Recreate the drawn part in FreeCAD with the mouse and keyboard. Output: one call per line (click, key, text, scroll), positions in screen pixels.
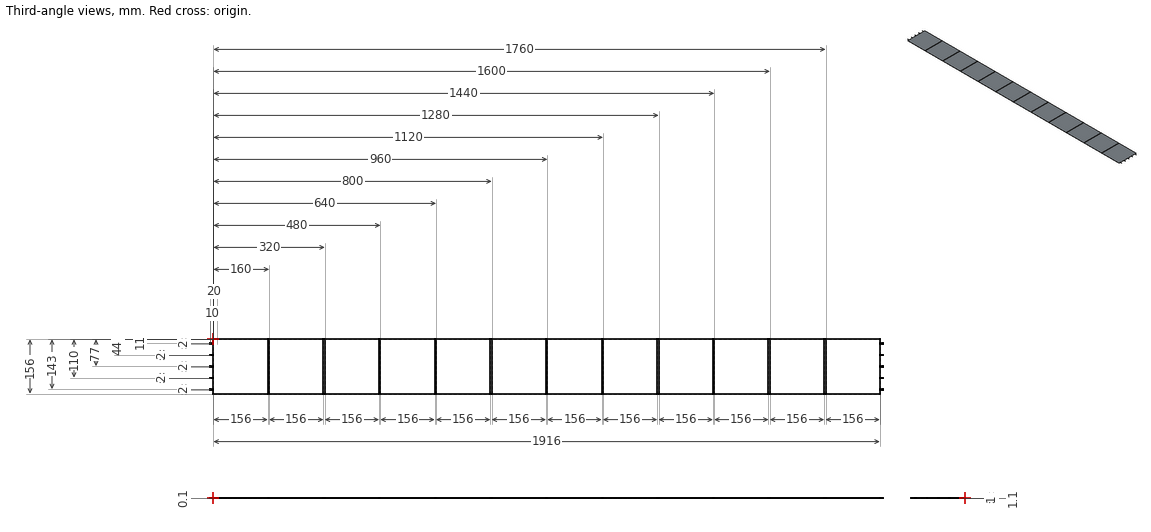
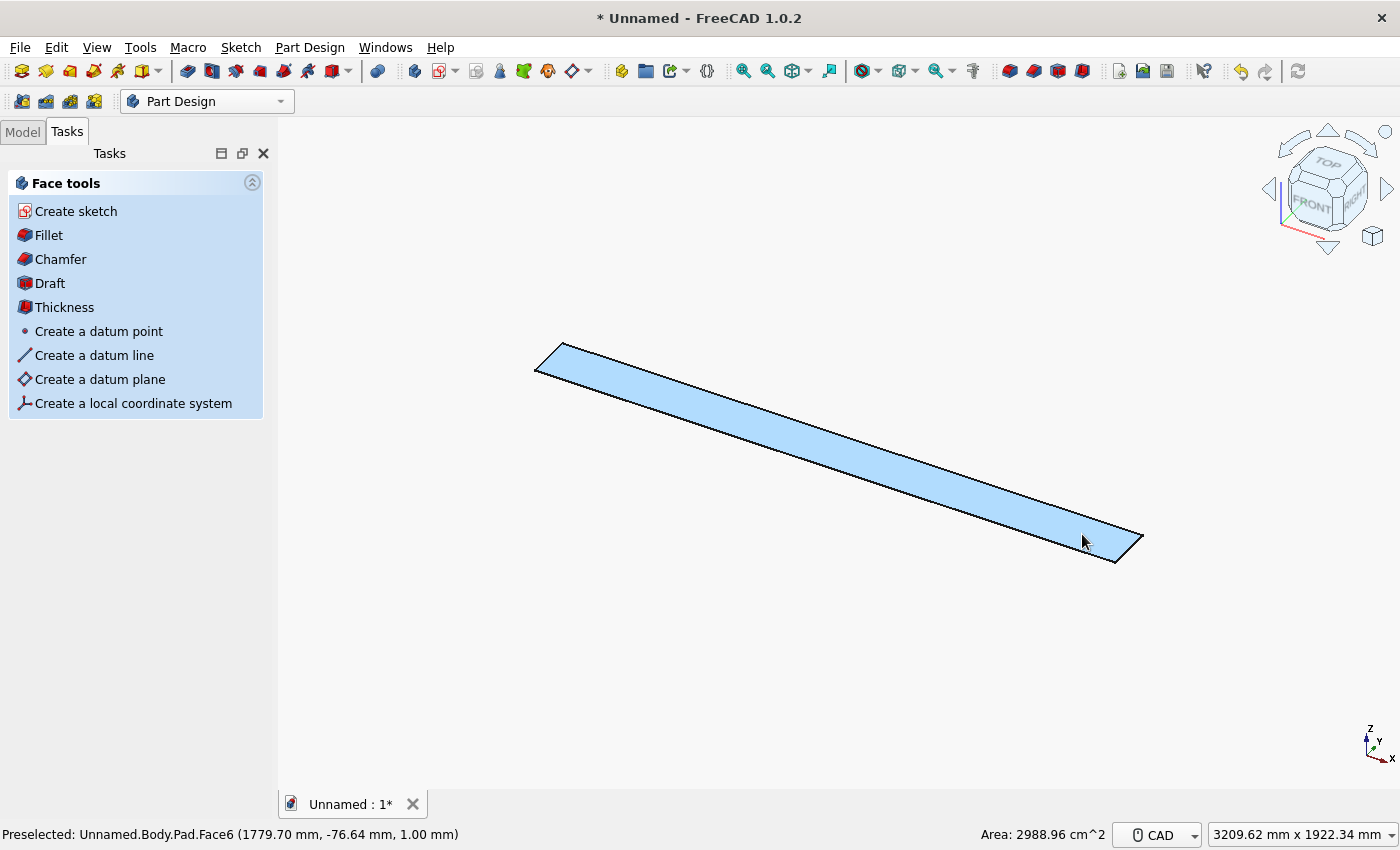
click(440, 72)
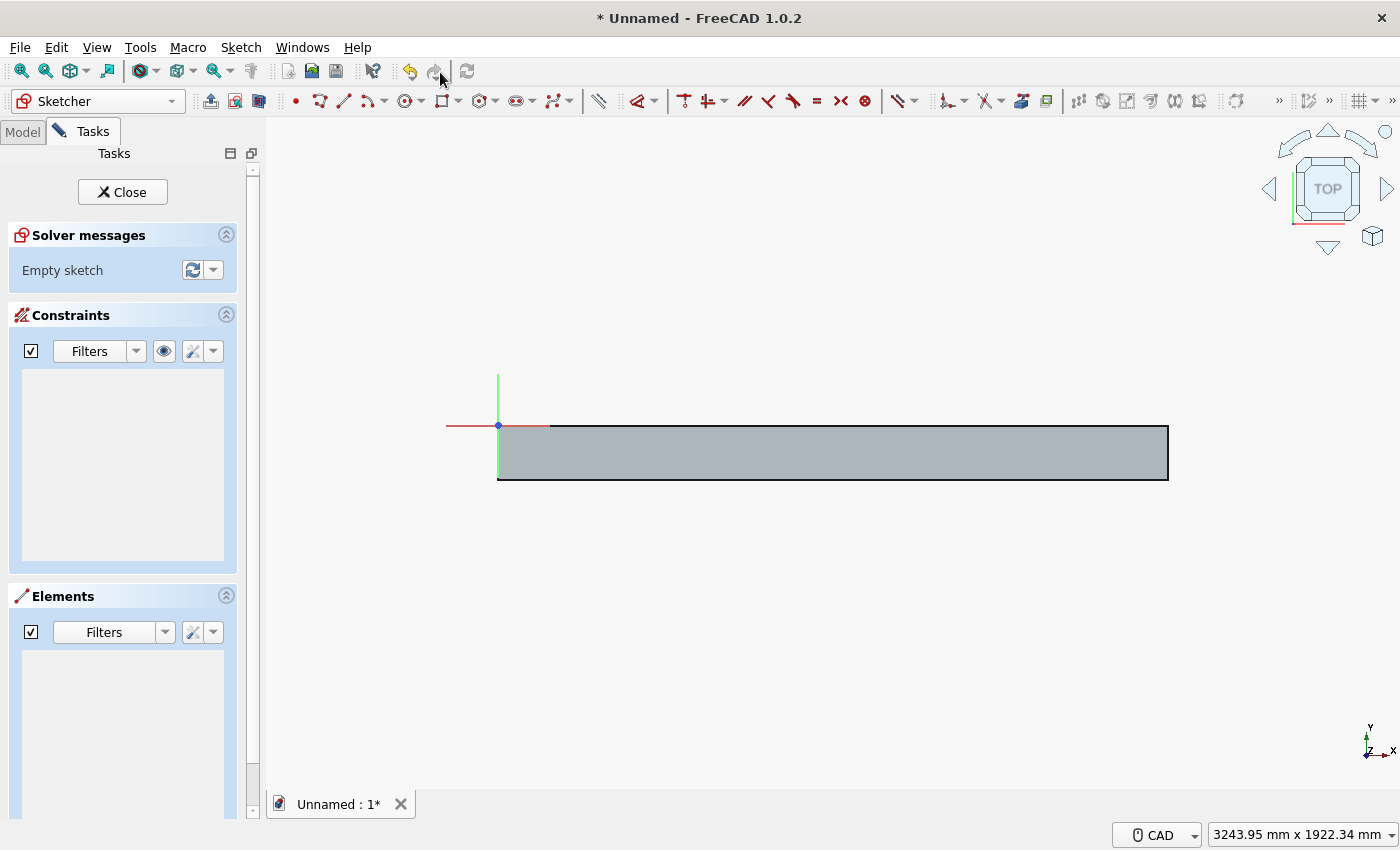
key(g)
key(r)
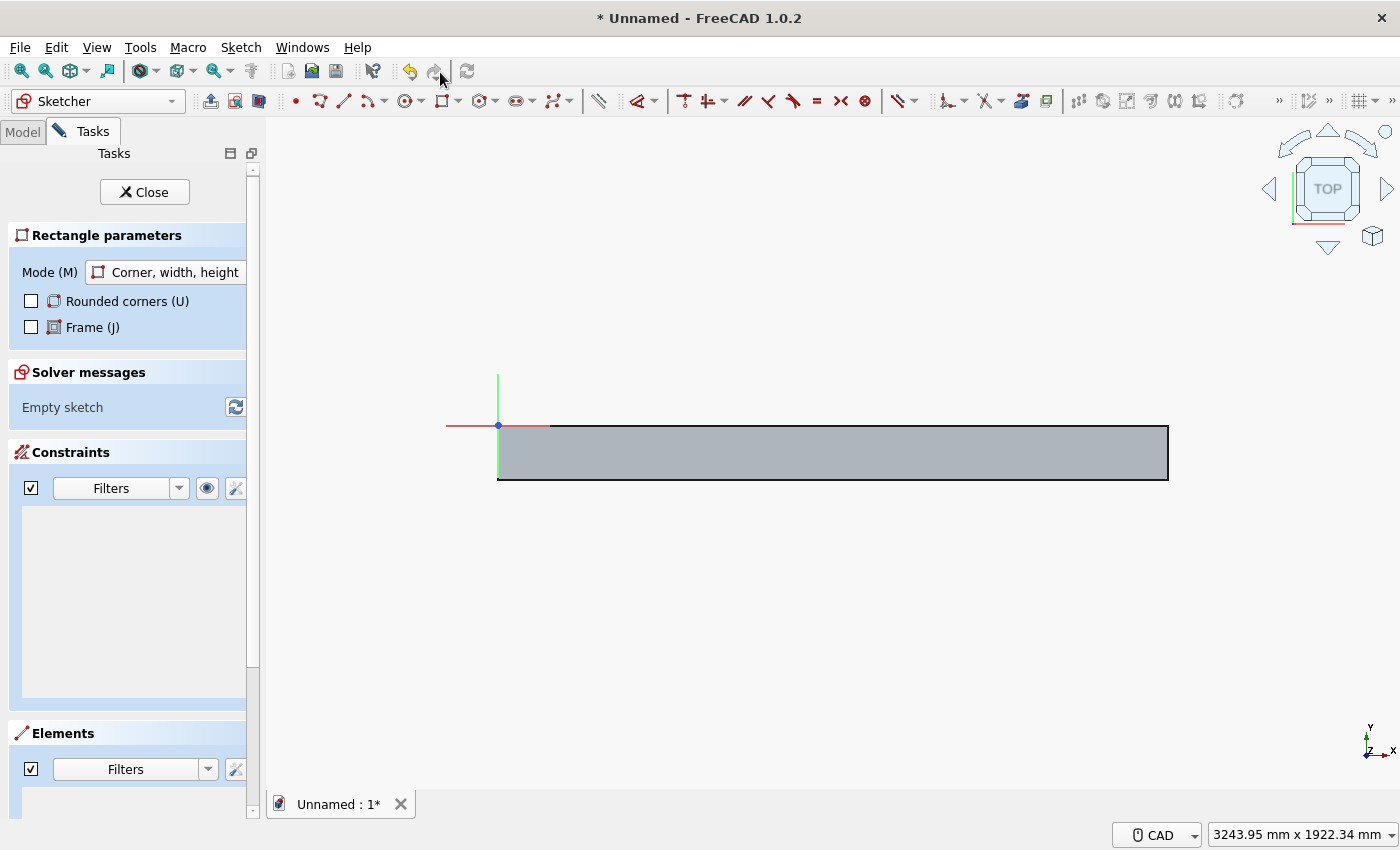
click(498, 426)
click(553, 480)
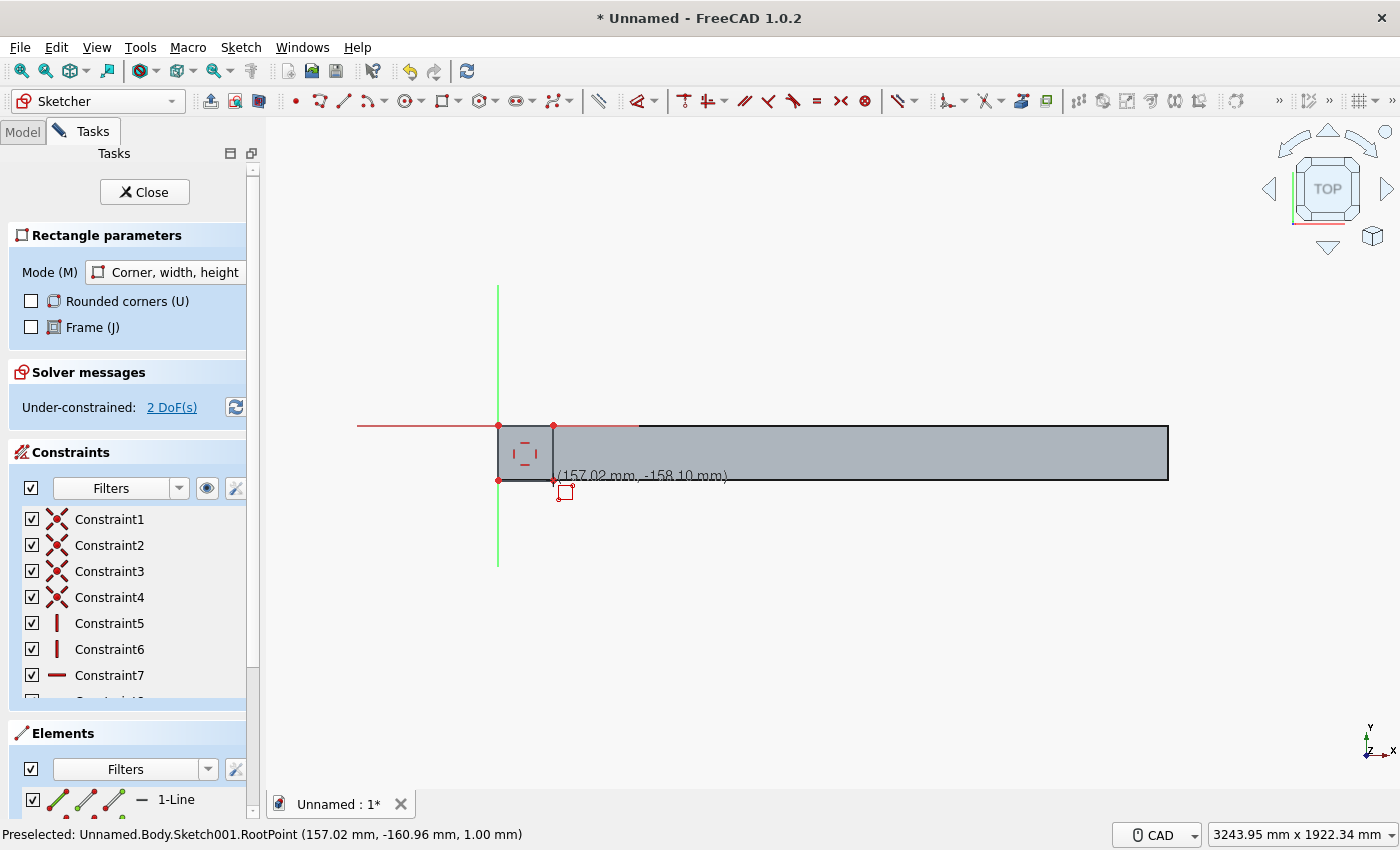
scroll(554, 426, up, 13)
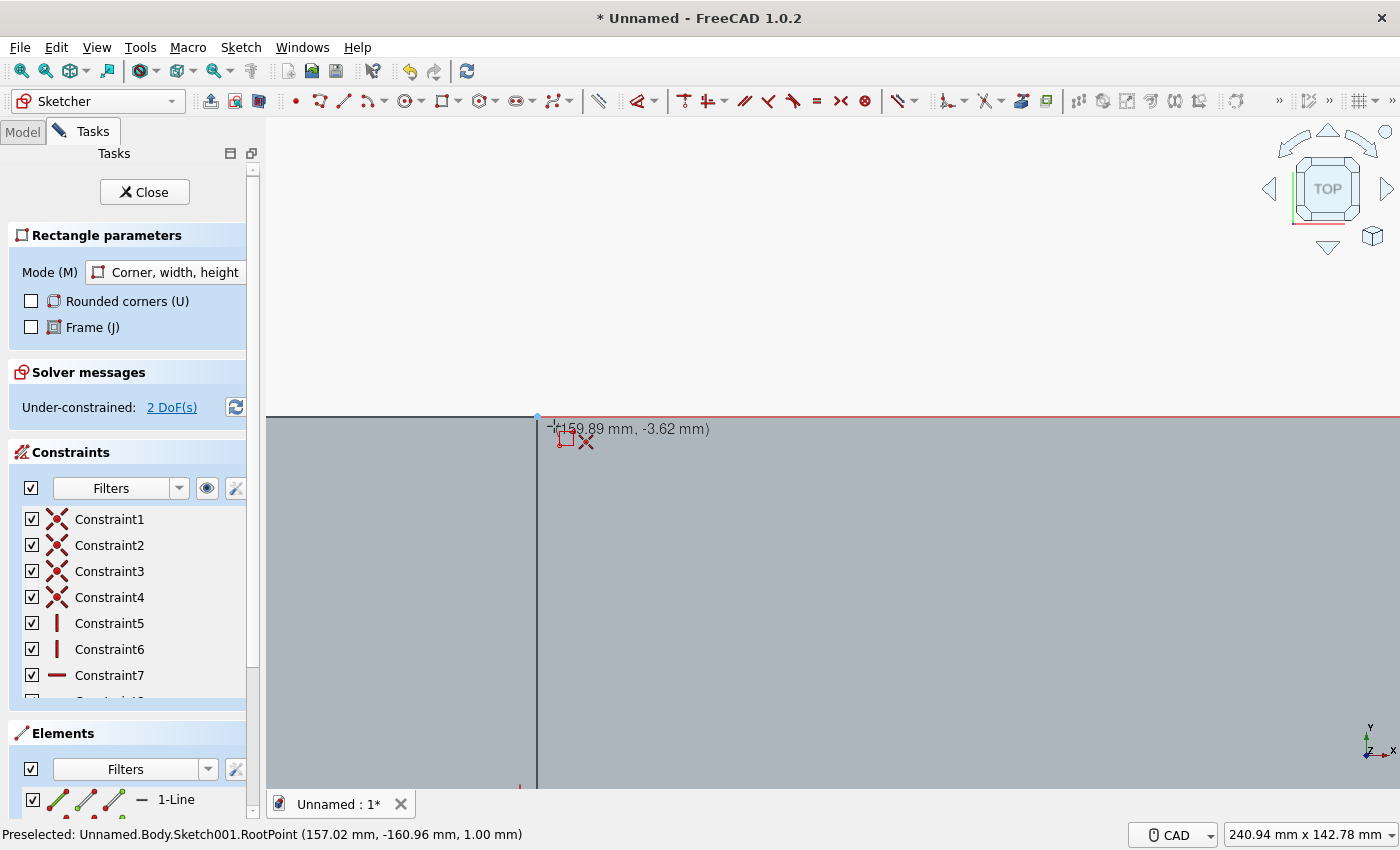
click(551, 417)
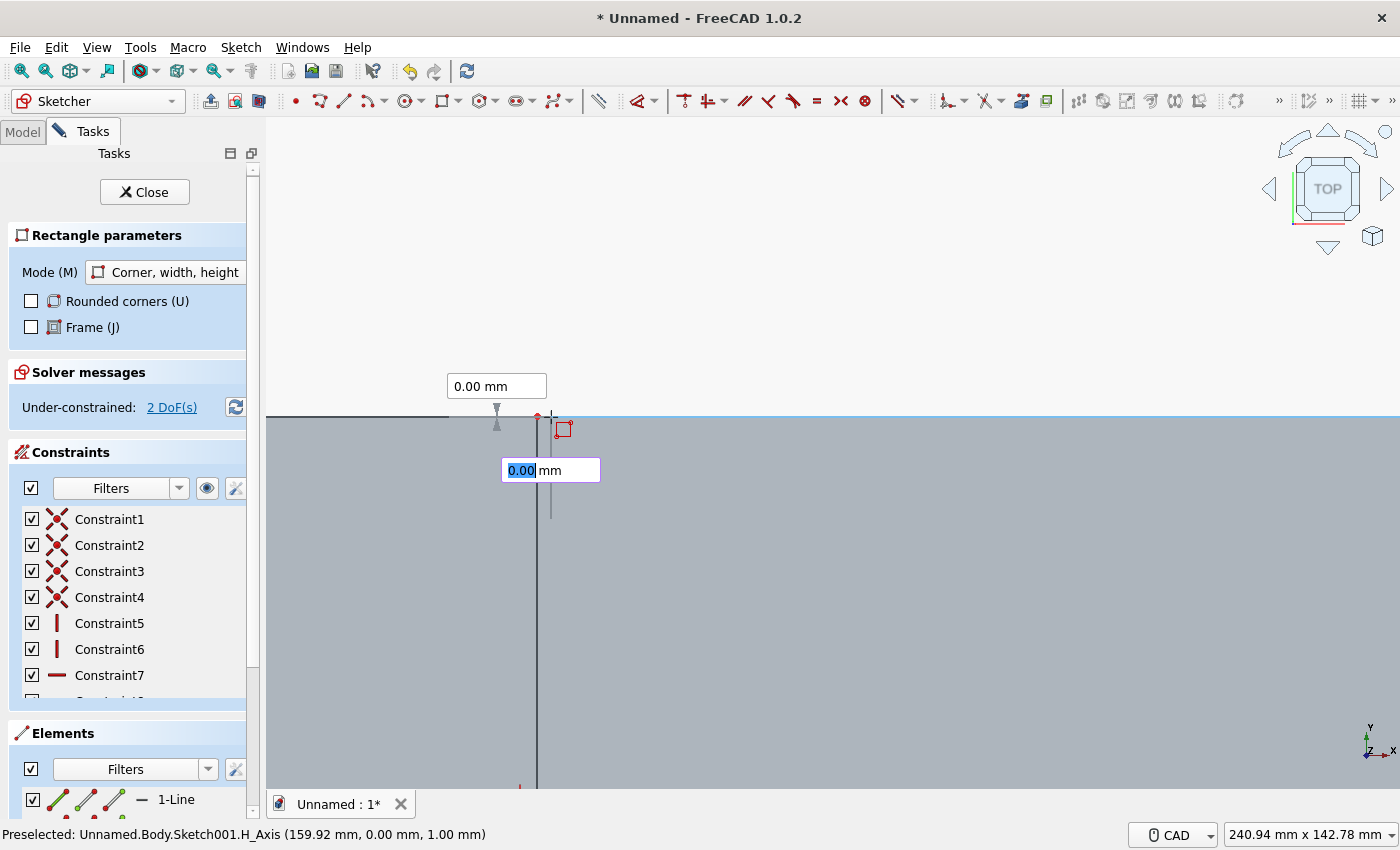
scroll(480, 426, down, 13)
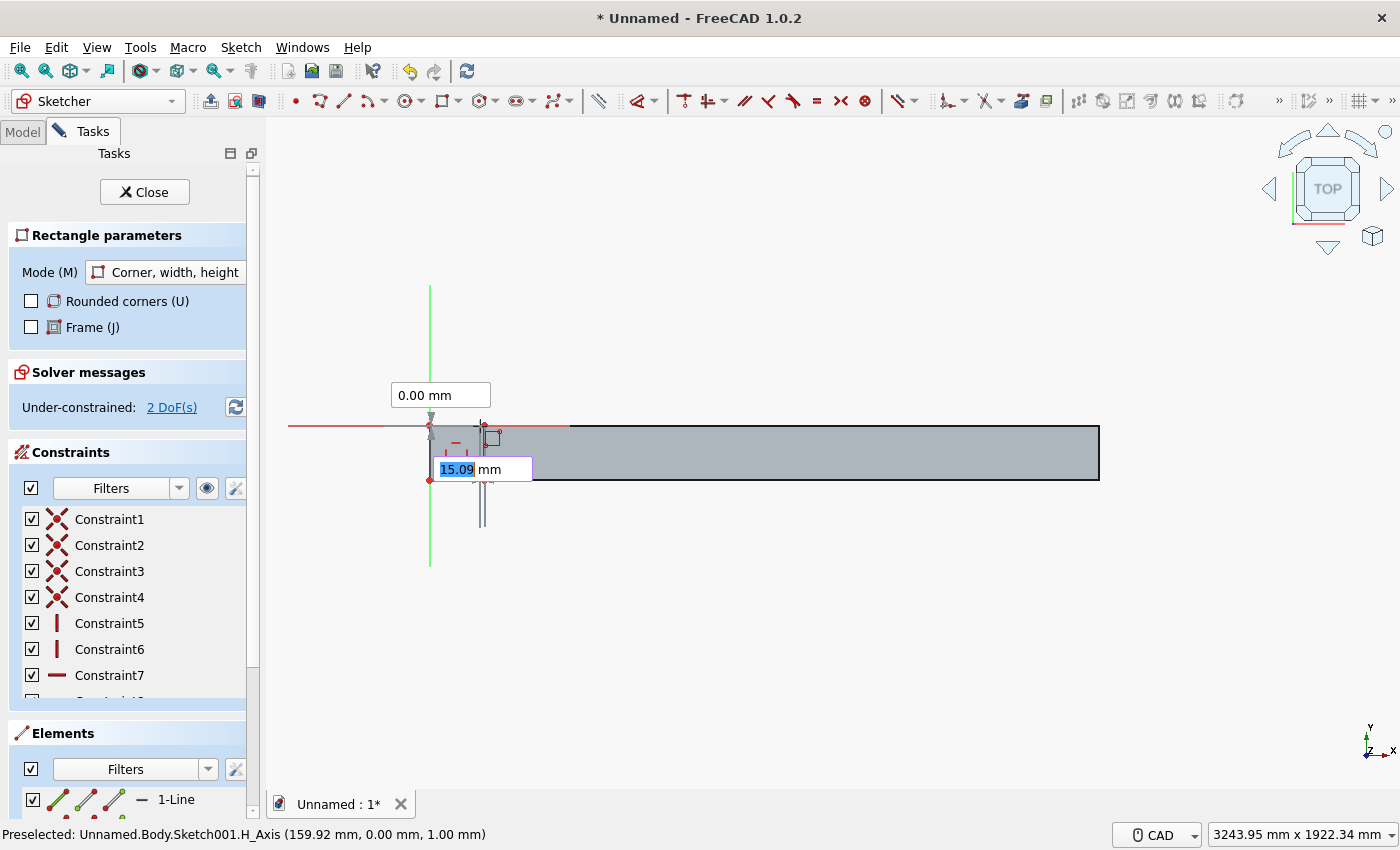
click(540, 480)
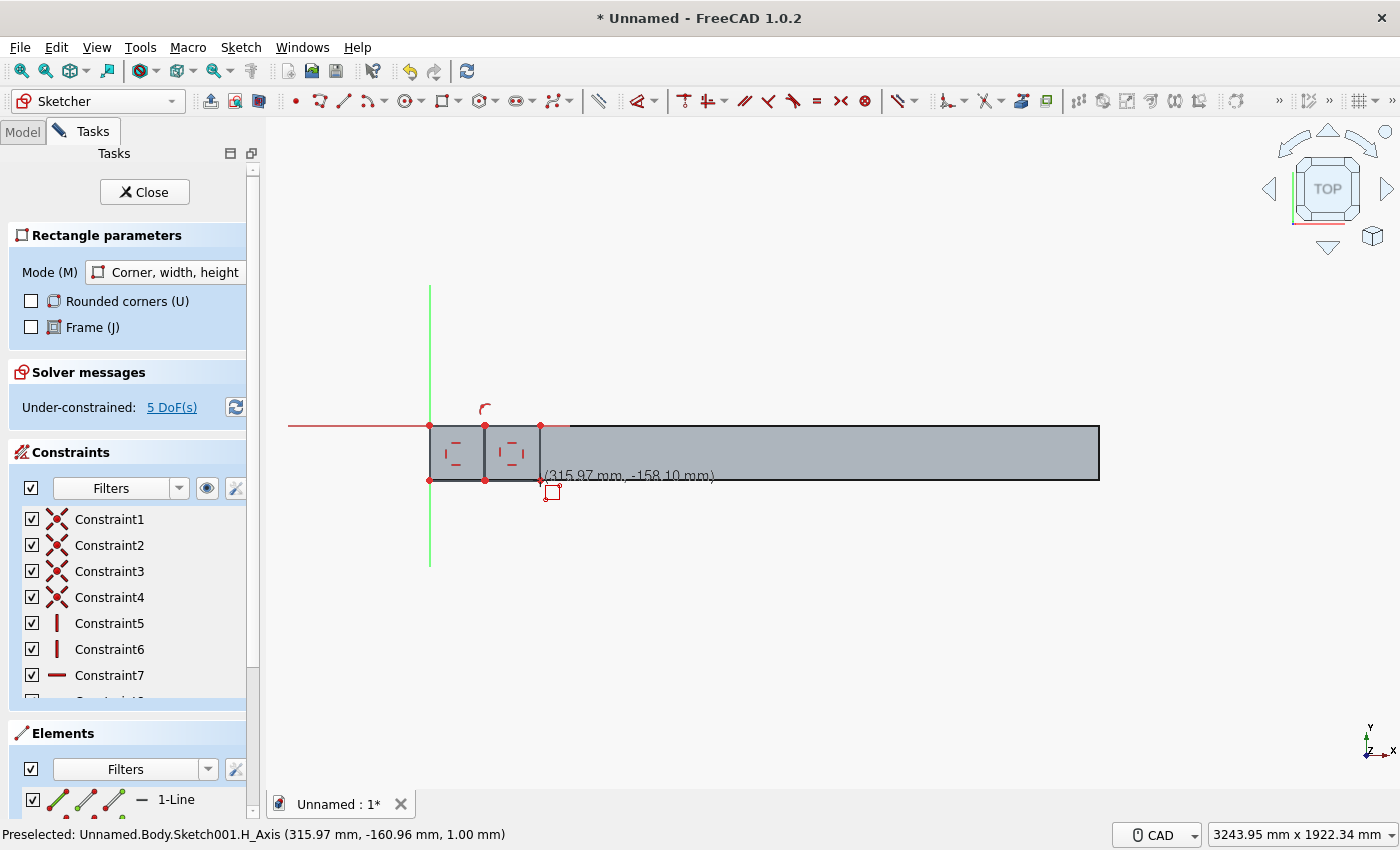
scroll(541, 426, up, 13)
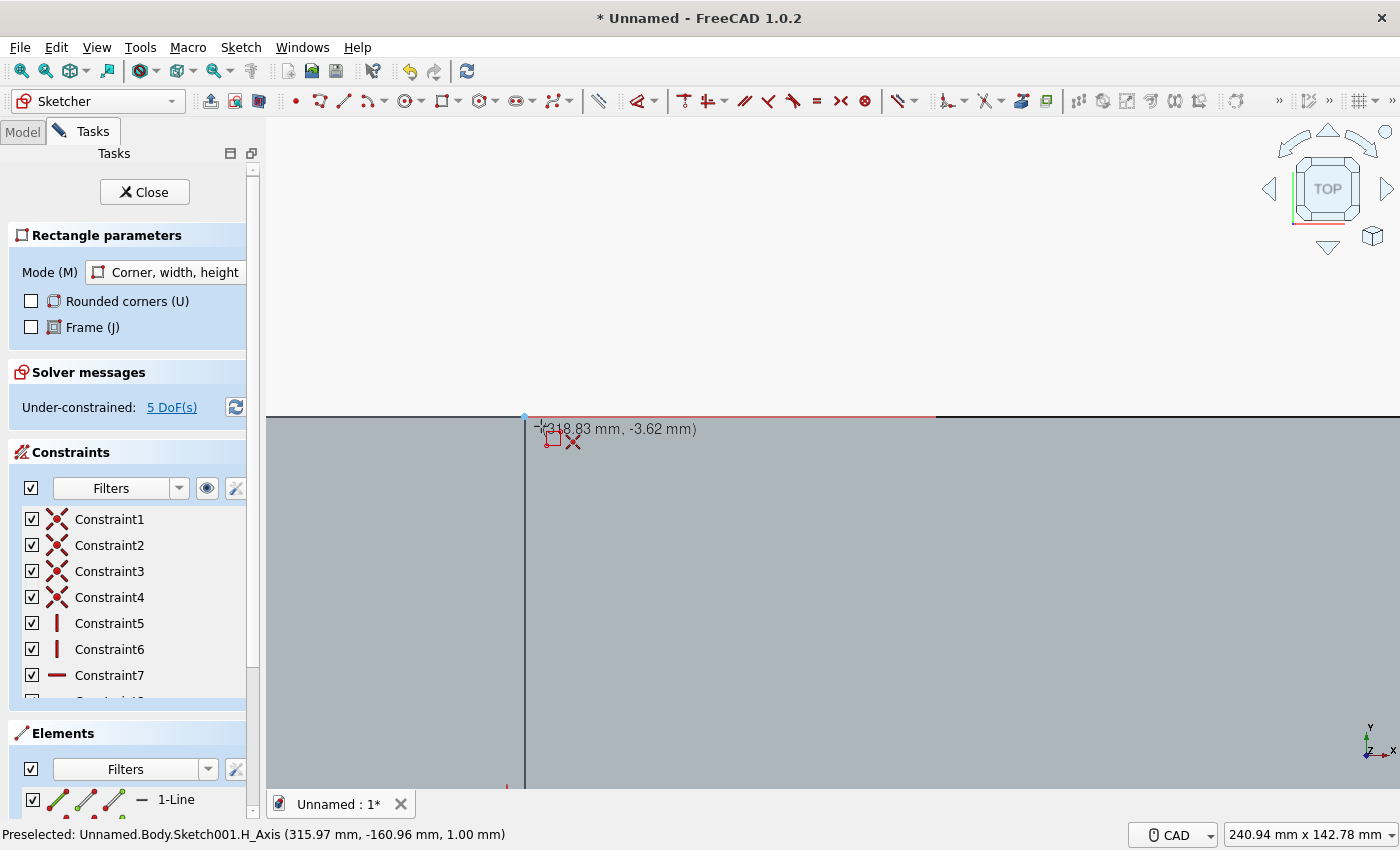
click(543, 417)